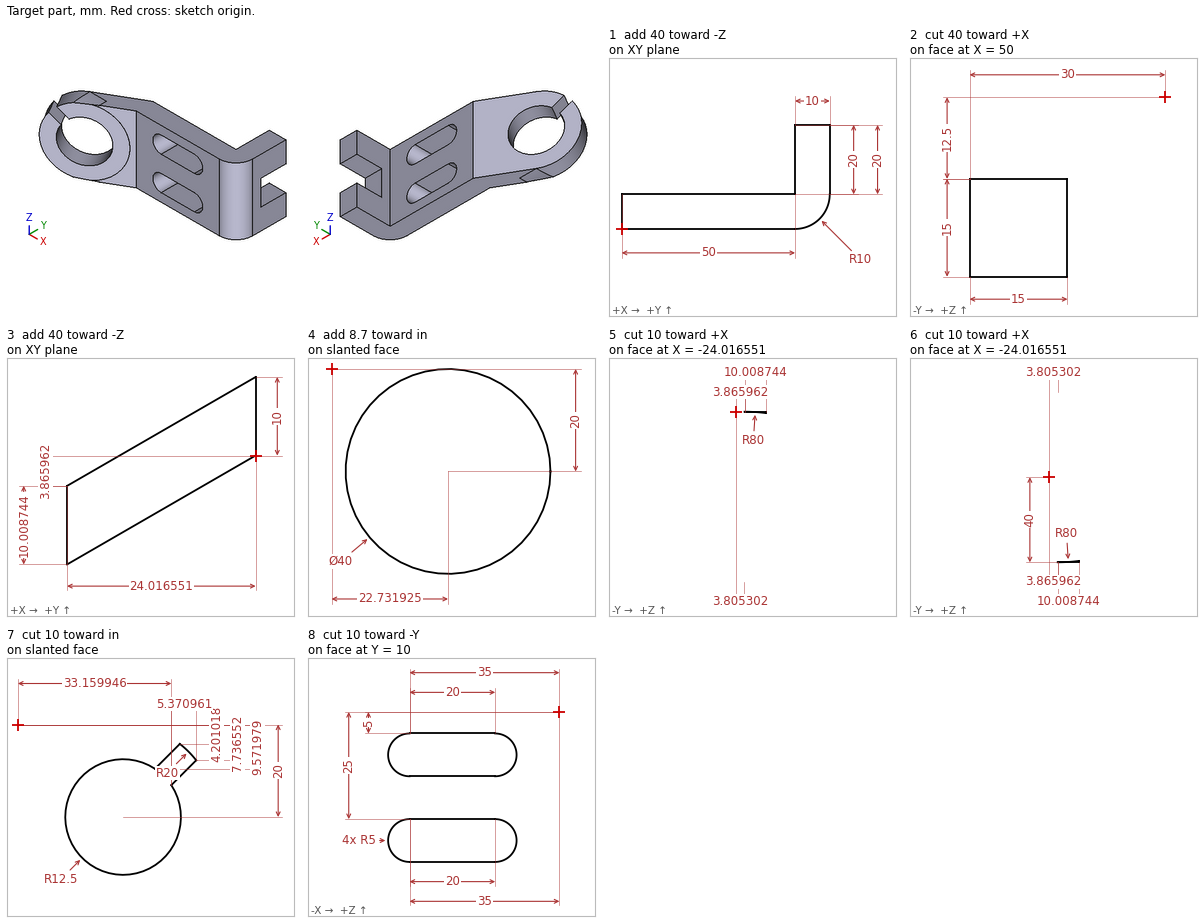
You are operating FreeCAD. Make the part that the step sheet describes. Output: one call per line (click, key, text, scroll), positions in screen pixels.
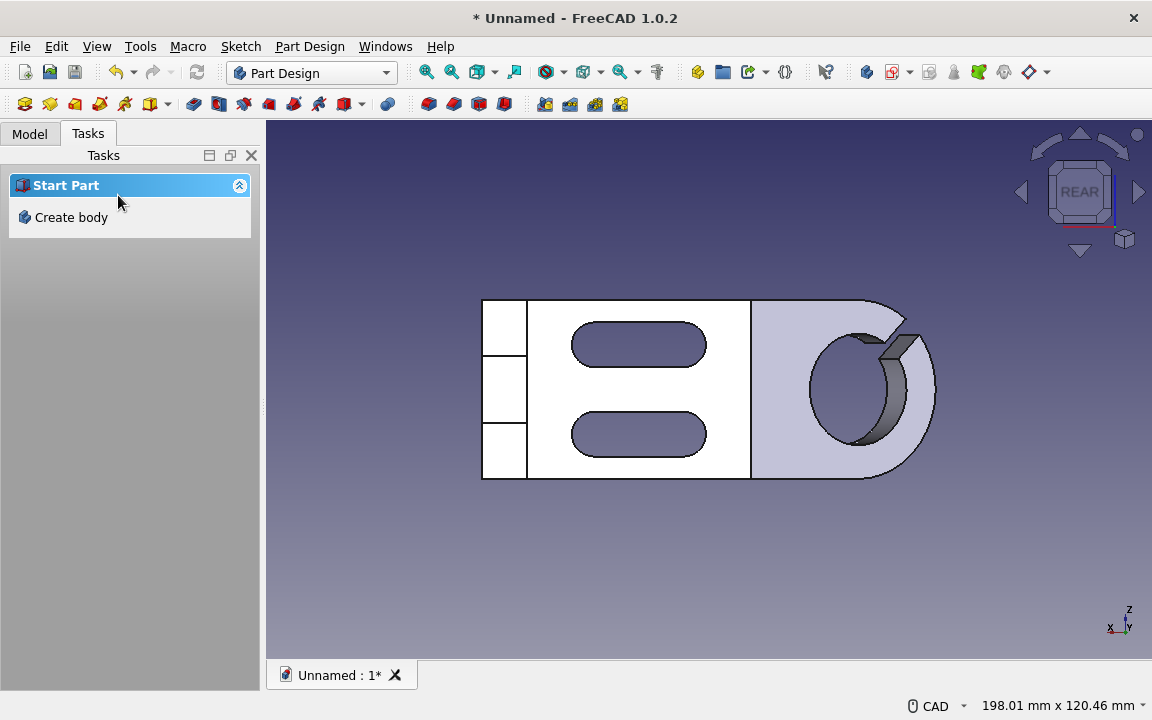
key(0)